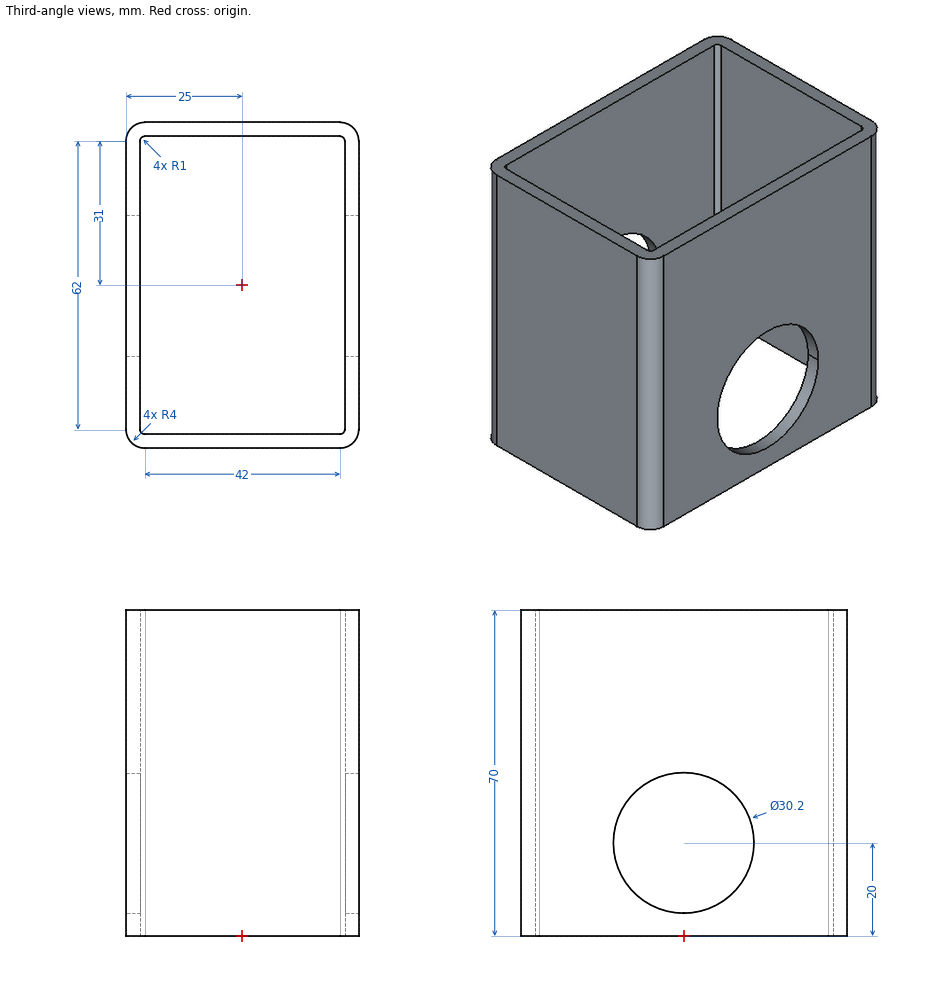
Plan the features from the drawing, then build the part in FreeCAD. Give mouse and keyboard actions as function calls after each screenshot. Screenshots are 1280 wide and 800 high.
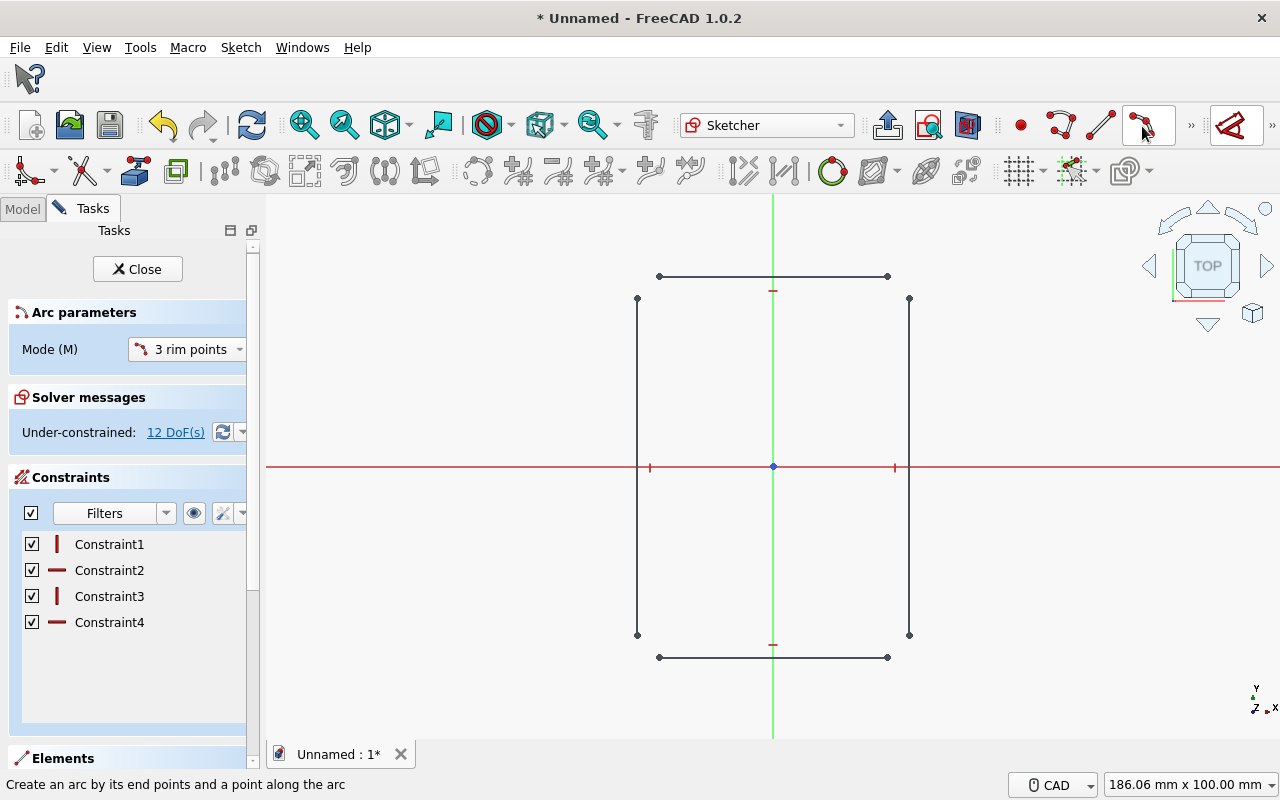
click(637, 636)
click(659, 658)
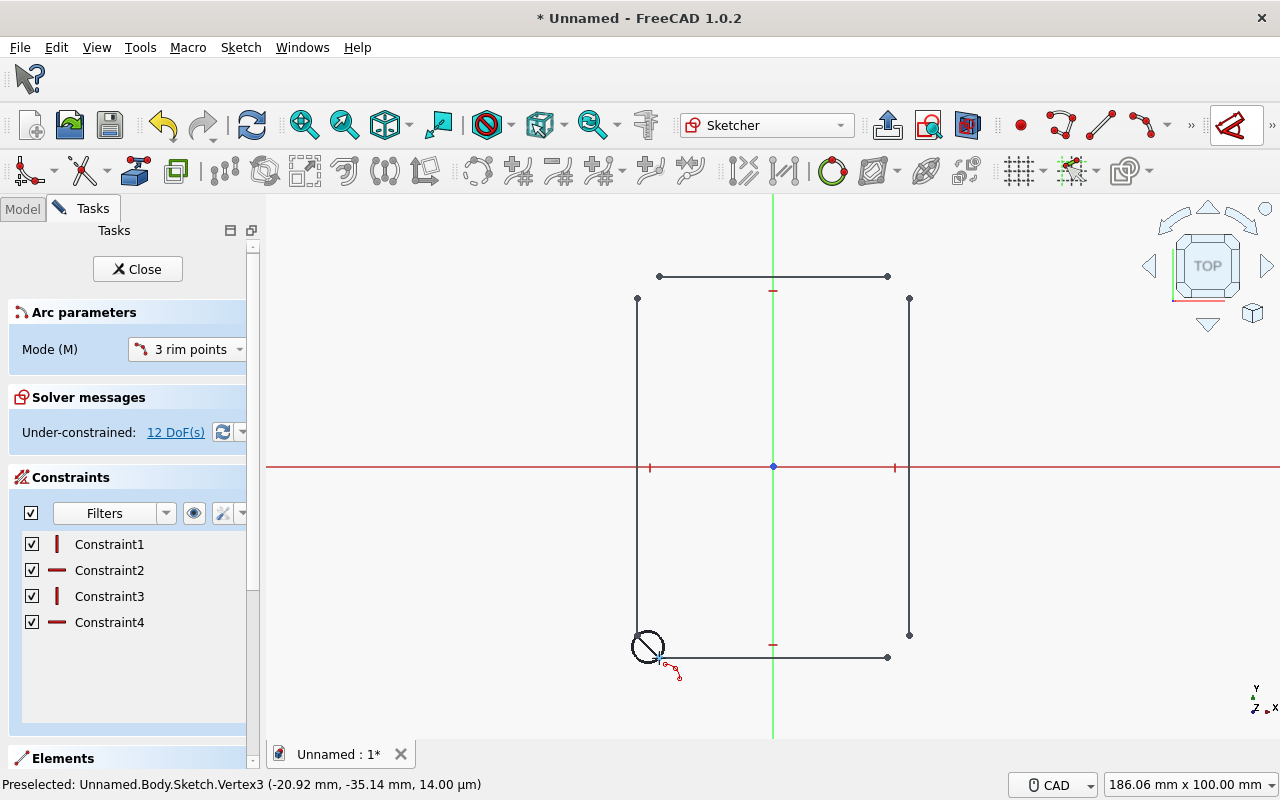
scroll(643, 651, up, 5)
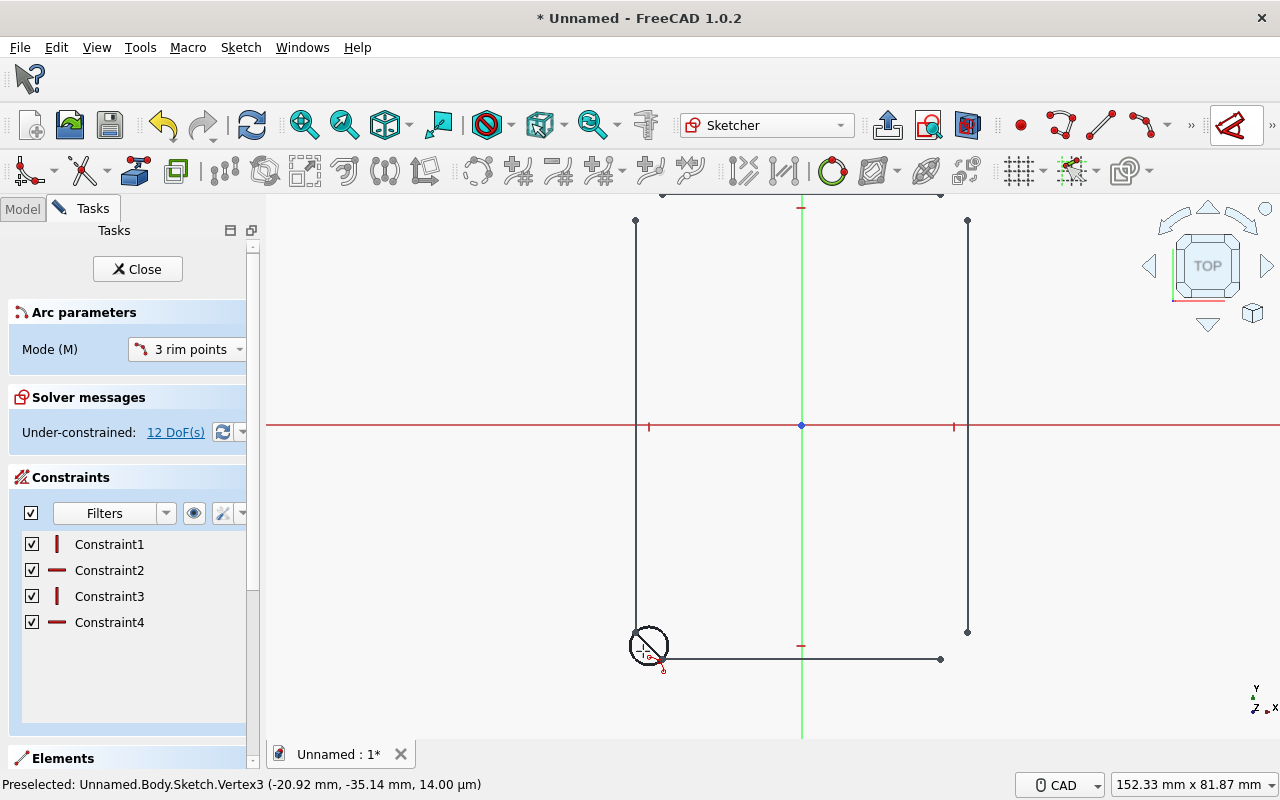
click(643, 649)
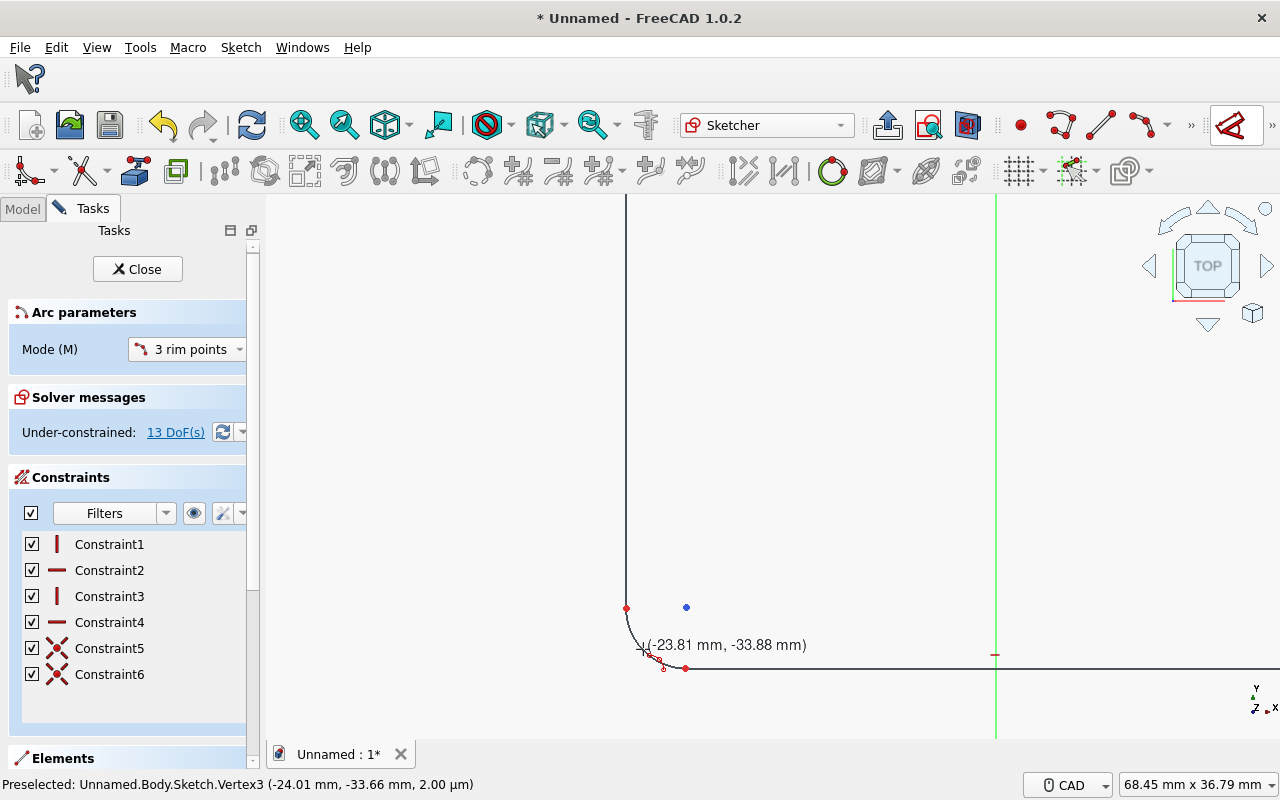
scroll(579, 604, down, 6)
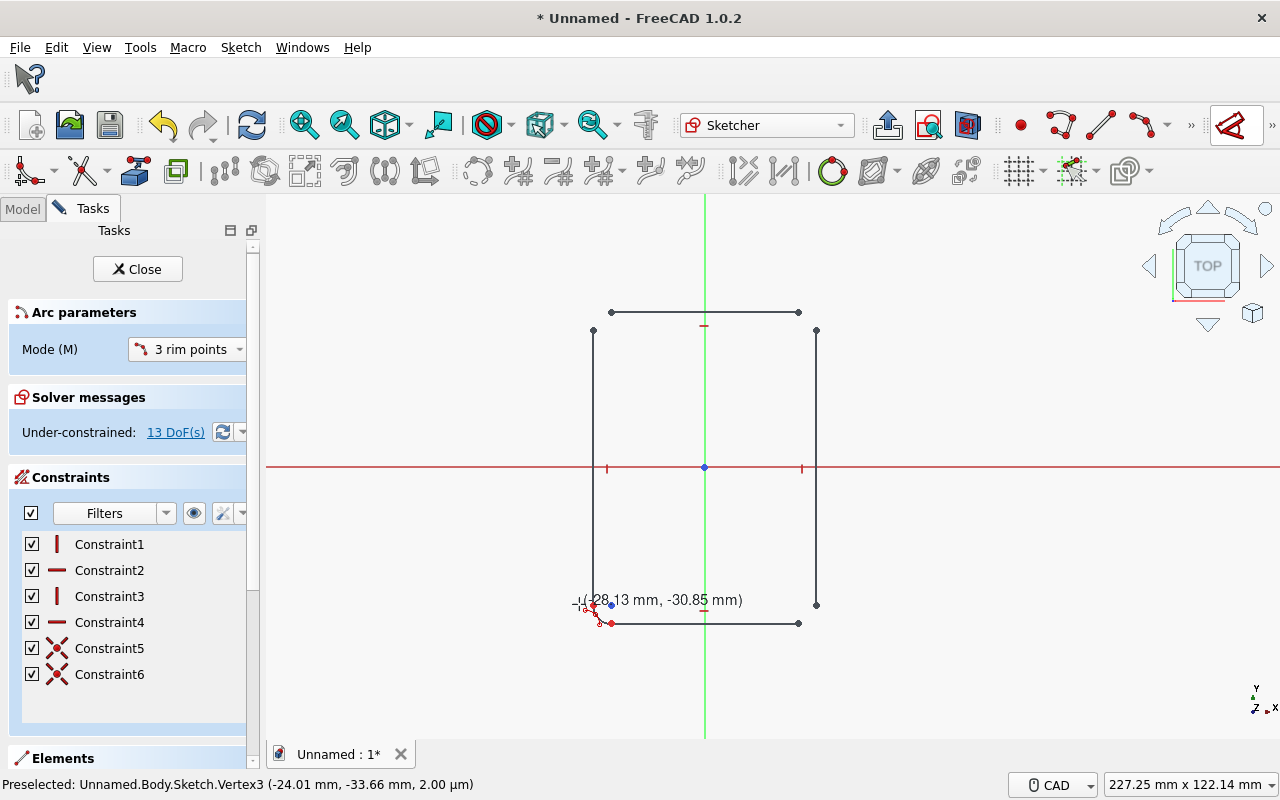
click(798, 624)
click(816, 606)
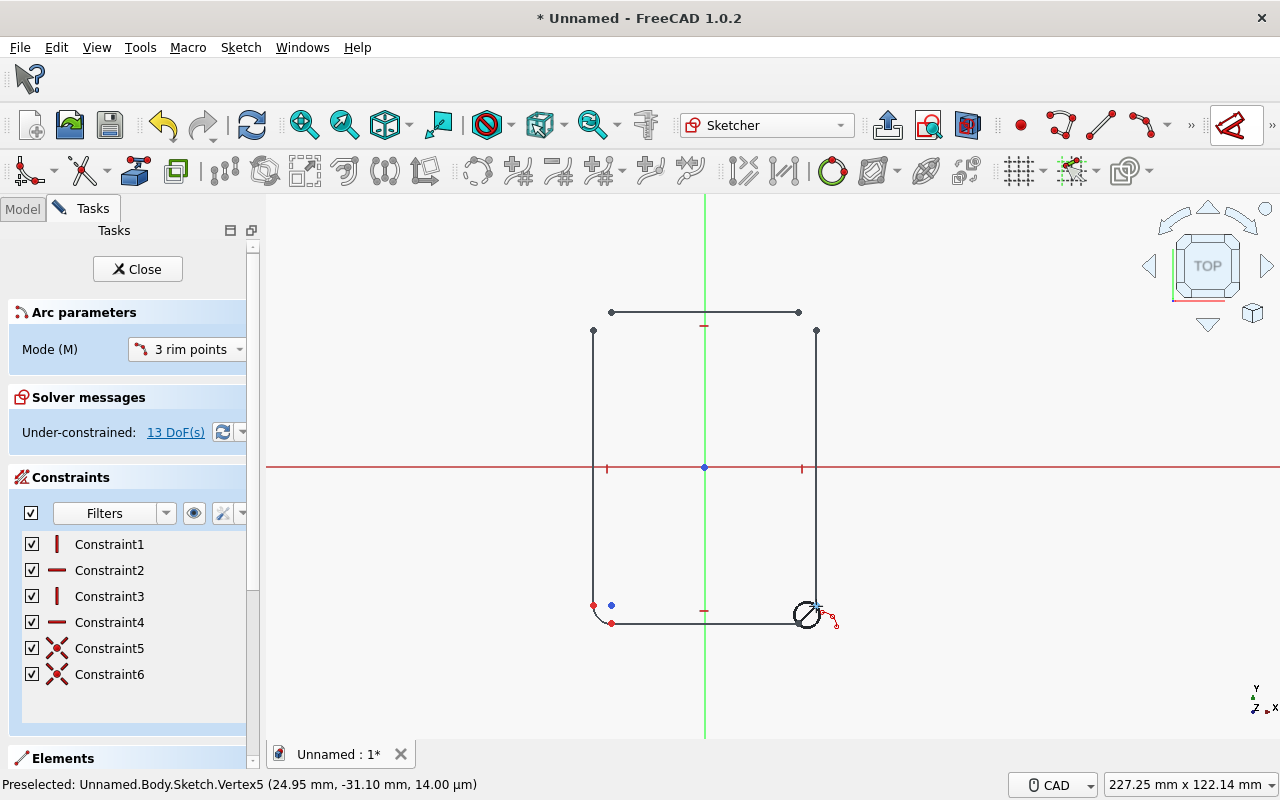
scroll(811, 618, up, 6)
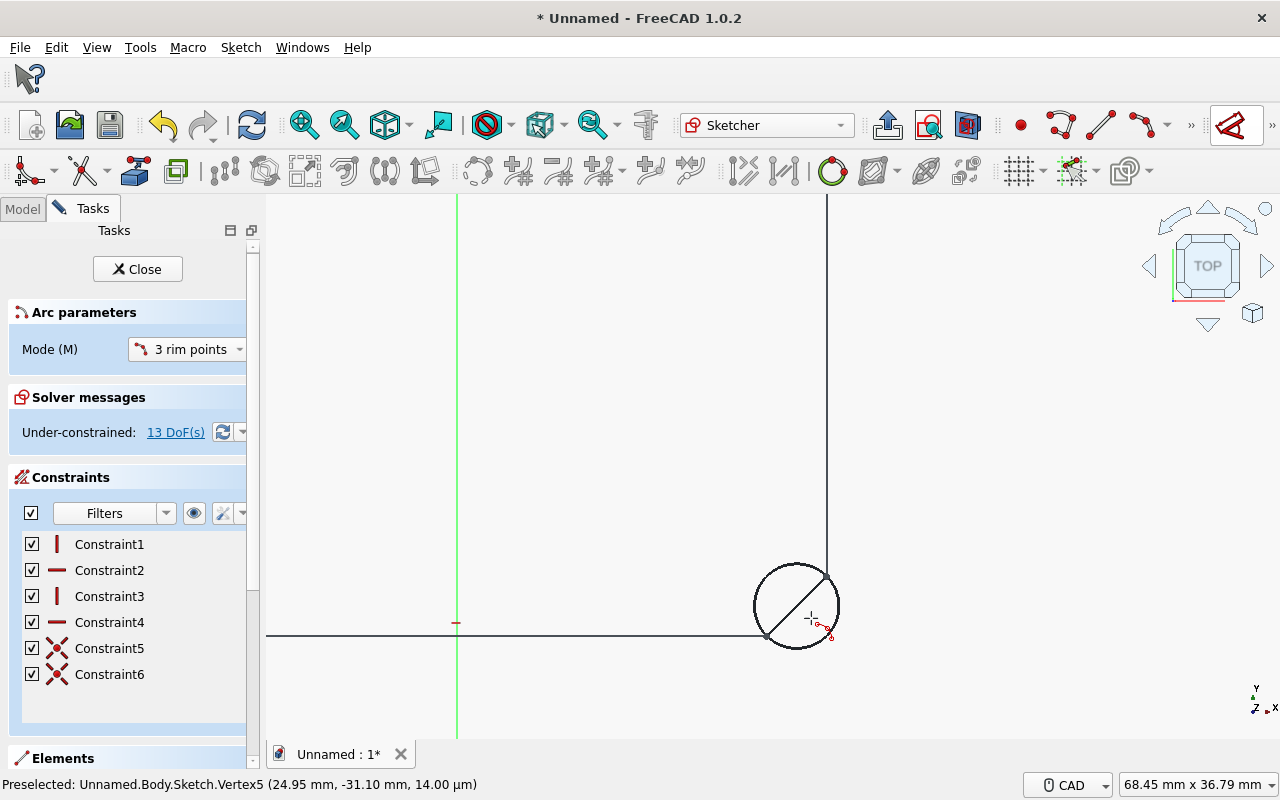
click(810, 617)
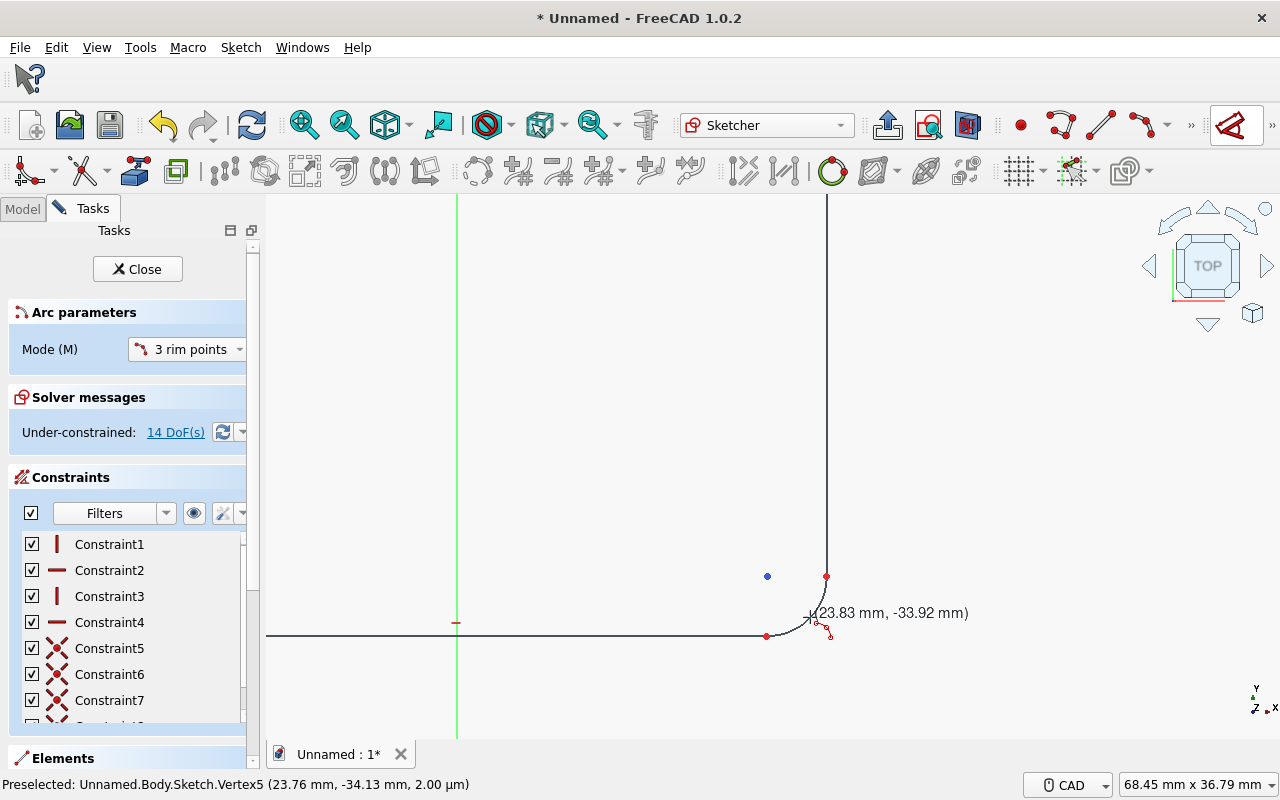
scroll(811, 618, down, 6)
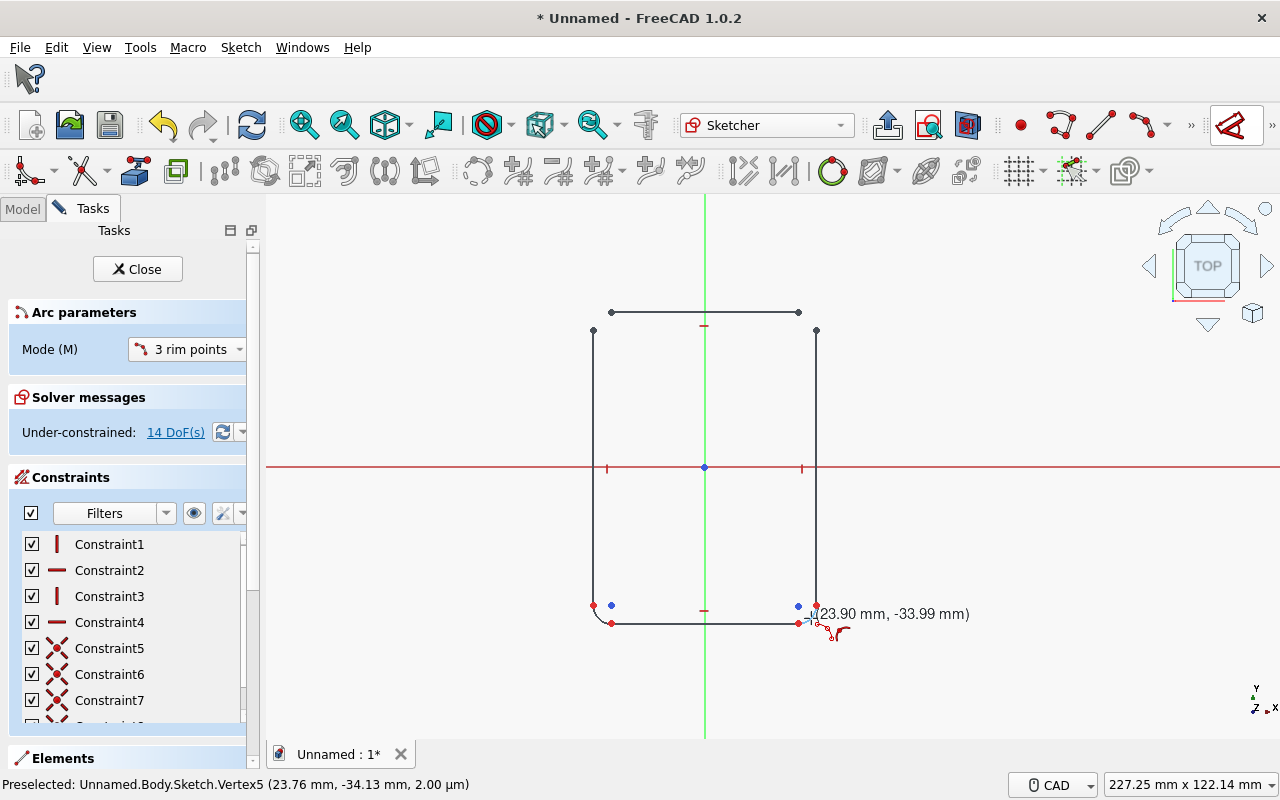
click(816, 330)
click(798, 312)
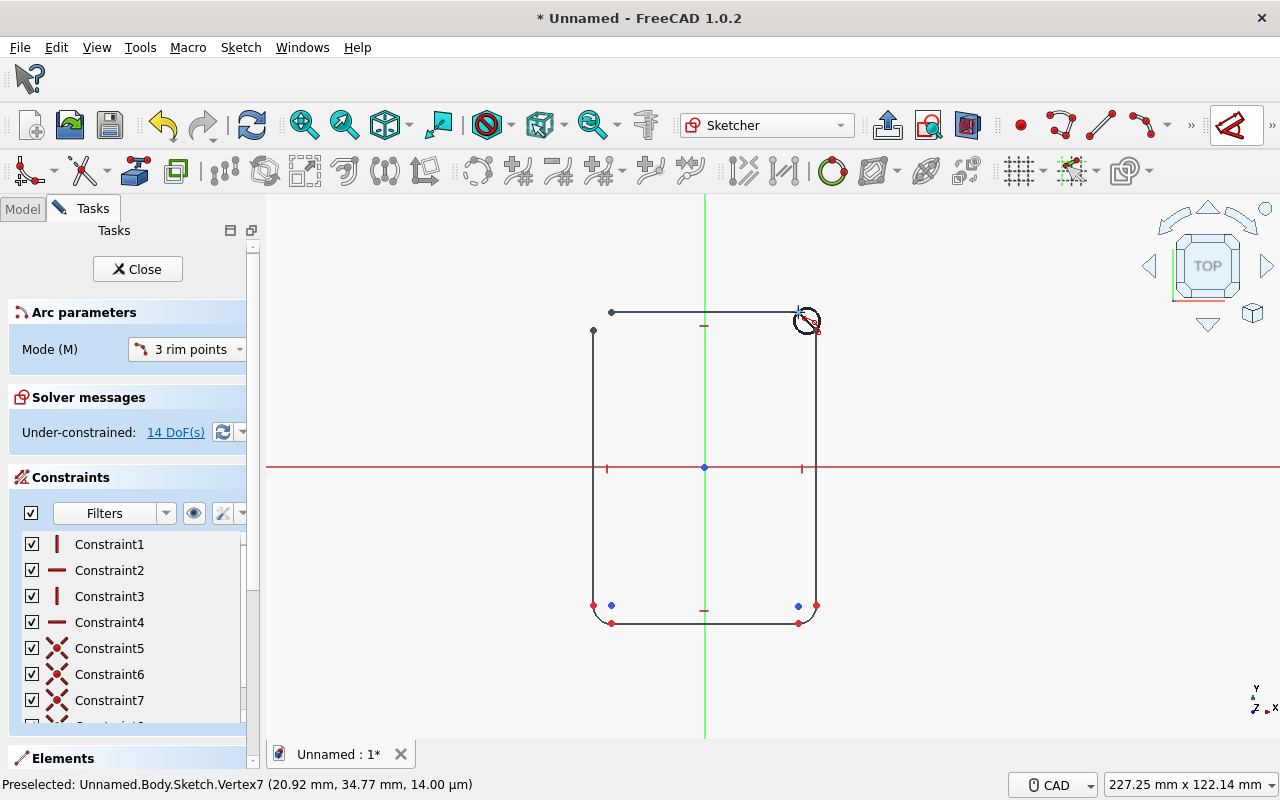
scroll(811, 316, up, 6)